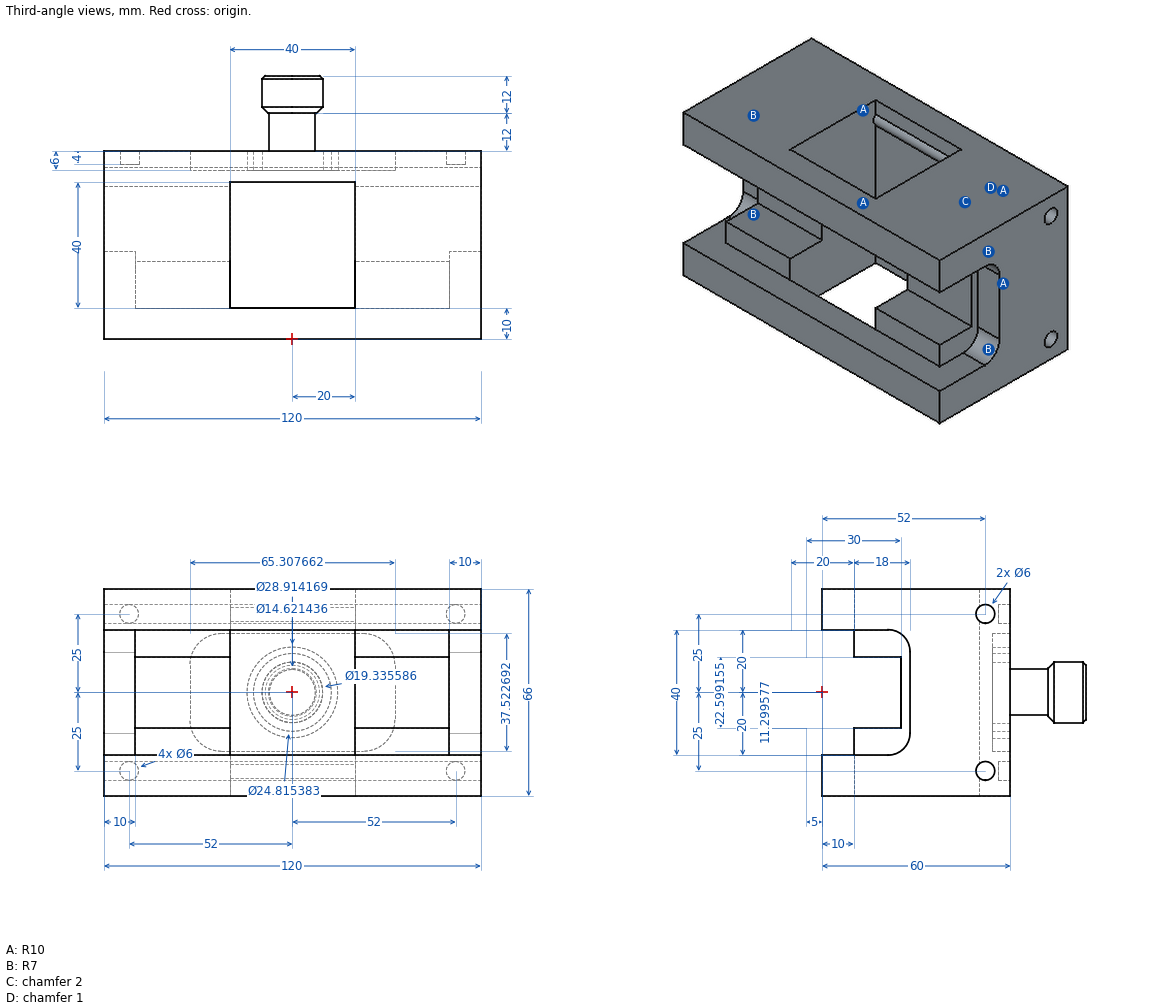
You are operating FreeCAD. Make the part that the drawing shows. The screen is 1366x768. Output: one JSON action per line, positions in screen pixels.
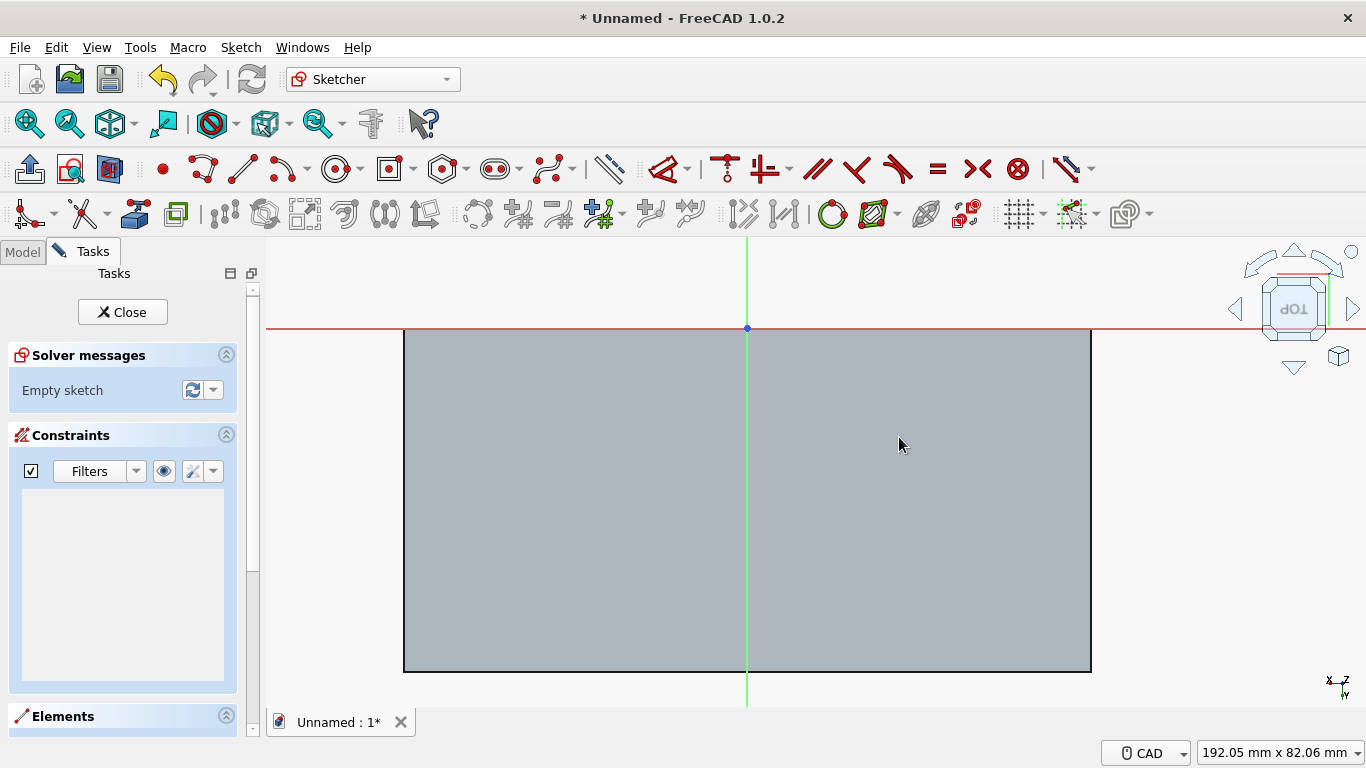
{"action": "key", "text": "g r"}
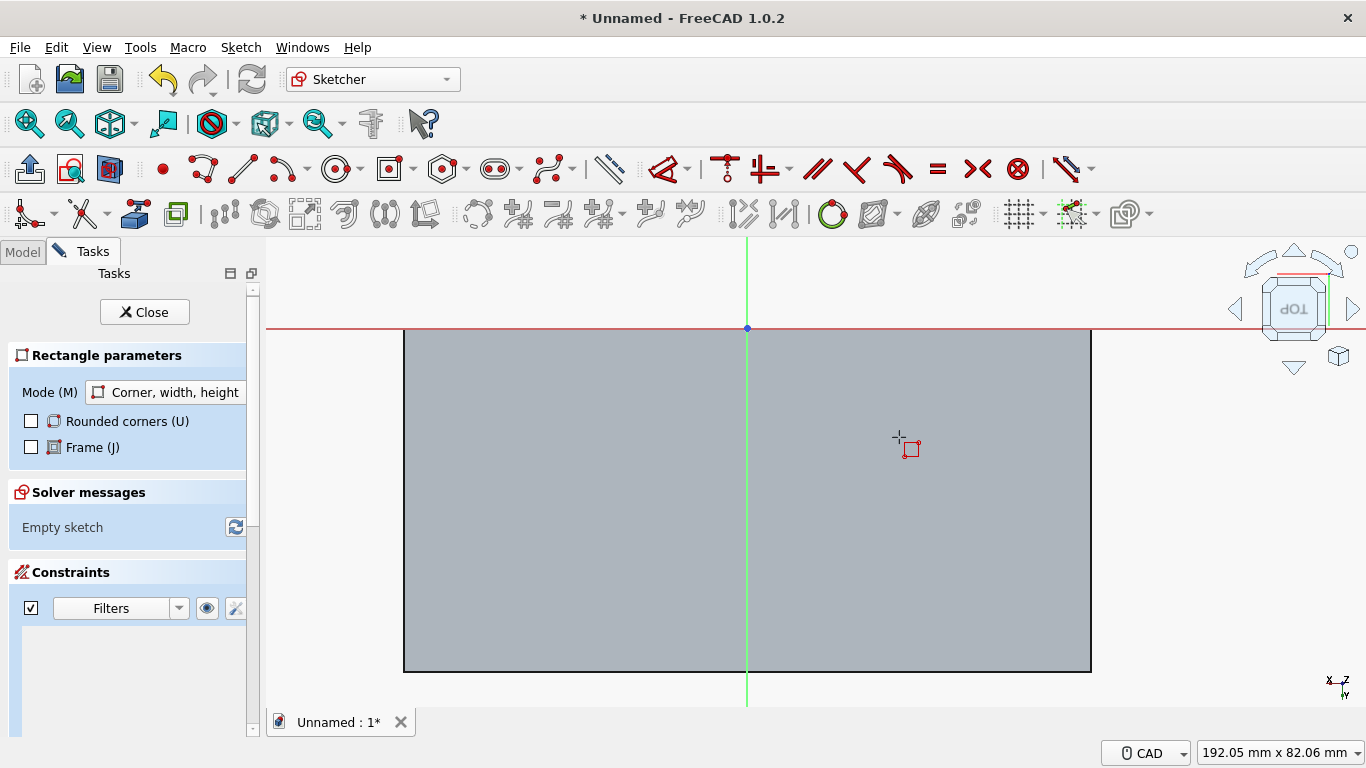
{"action": "left_click", "coordinate": [633, 386]}
{"action": "mouse_move", "coordinate": [862, 615]}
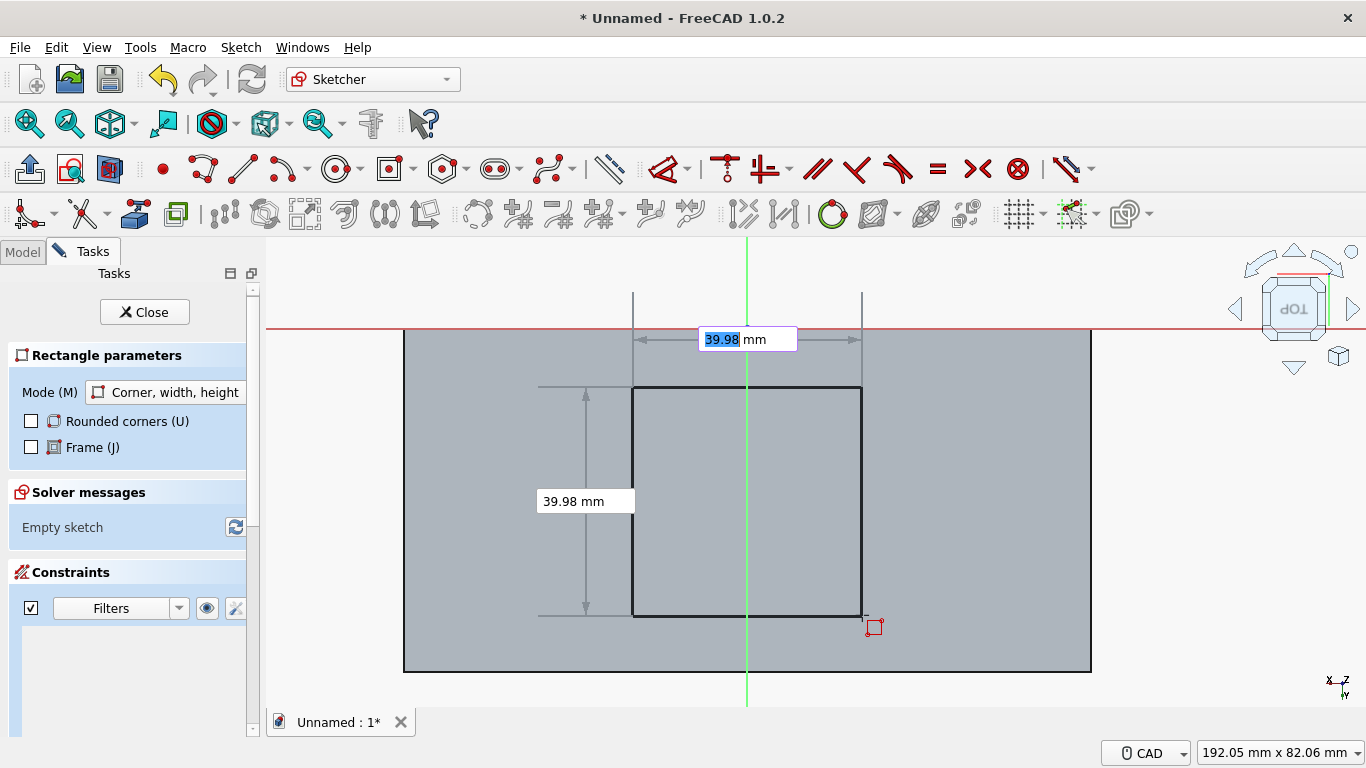
{"action": "type", "text": "40"}
{"action": "key", "text": "Tab"}
{"action": "type", "text": "40"}
{"action": "key", "text": "Return"}
{"action": "key", "text": "Escape"}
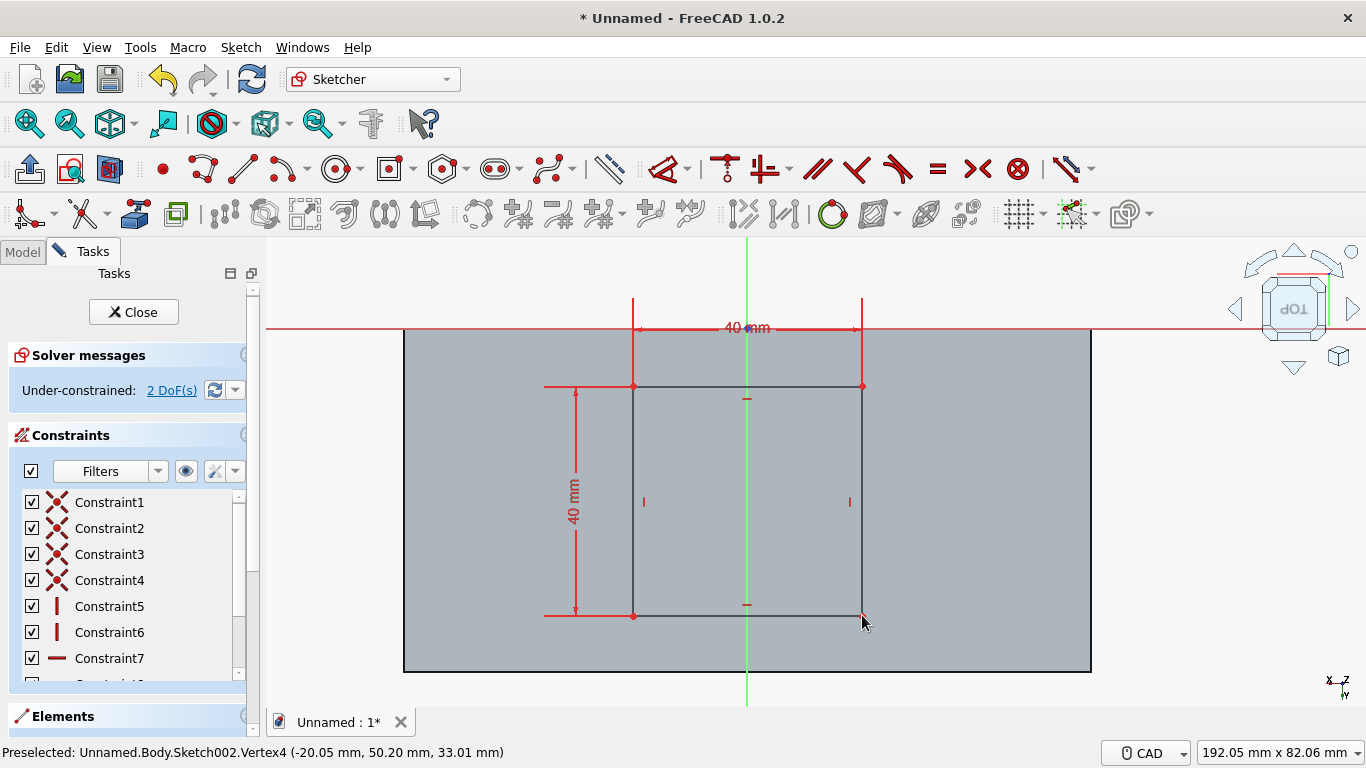
{"action": "left_click", "coordinate": [664, 170]}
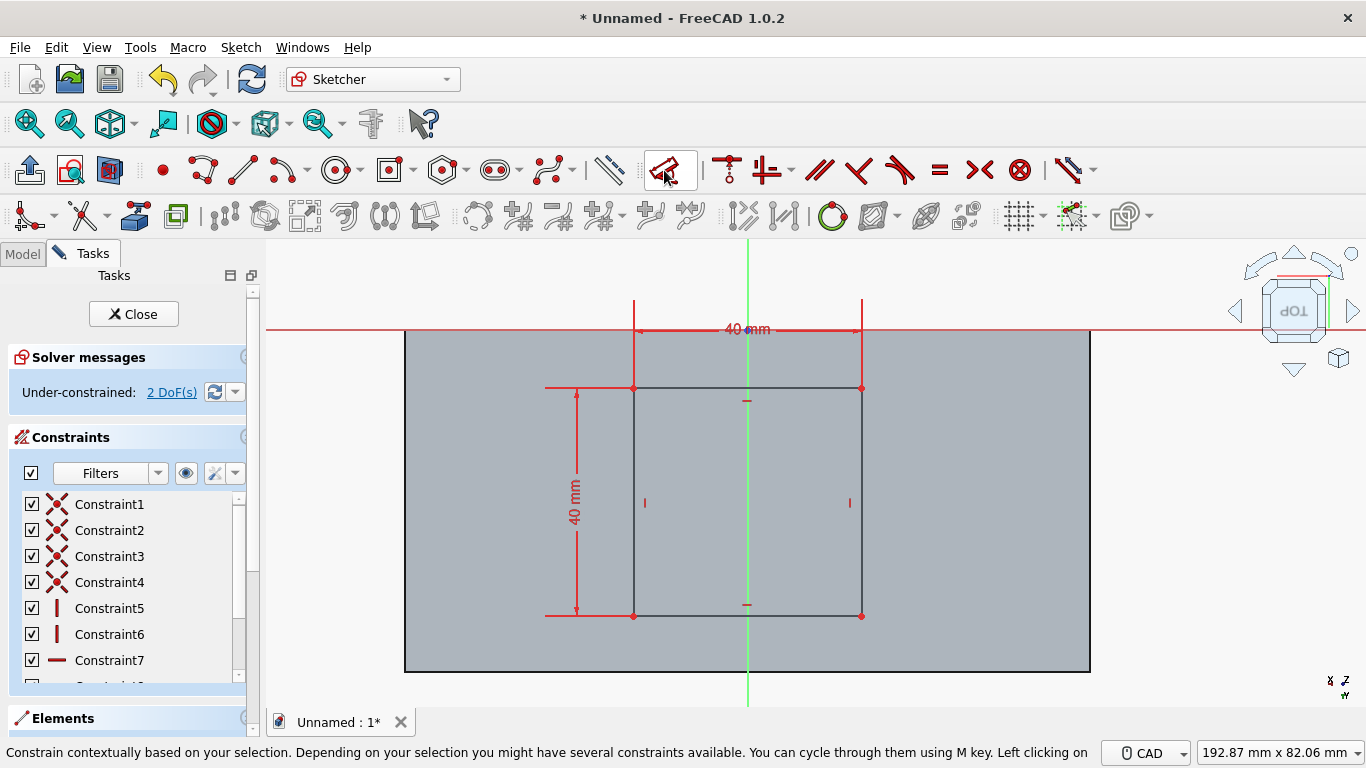
{"action": "left_click", "coordinate": [634, 388]}
{"action": "left_click", "coordinate": [691, 296]}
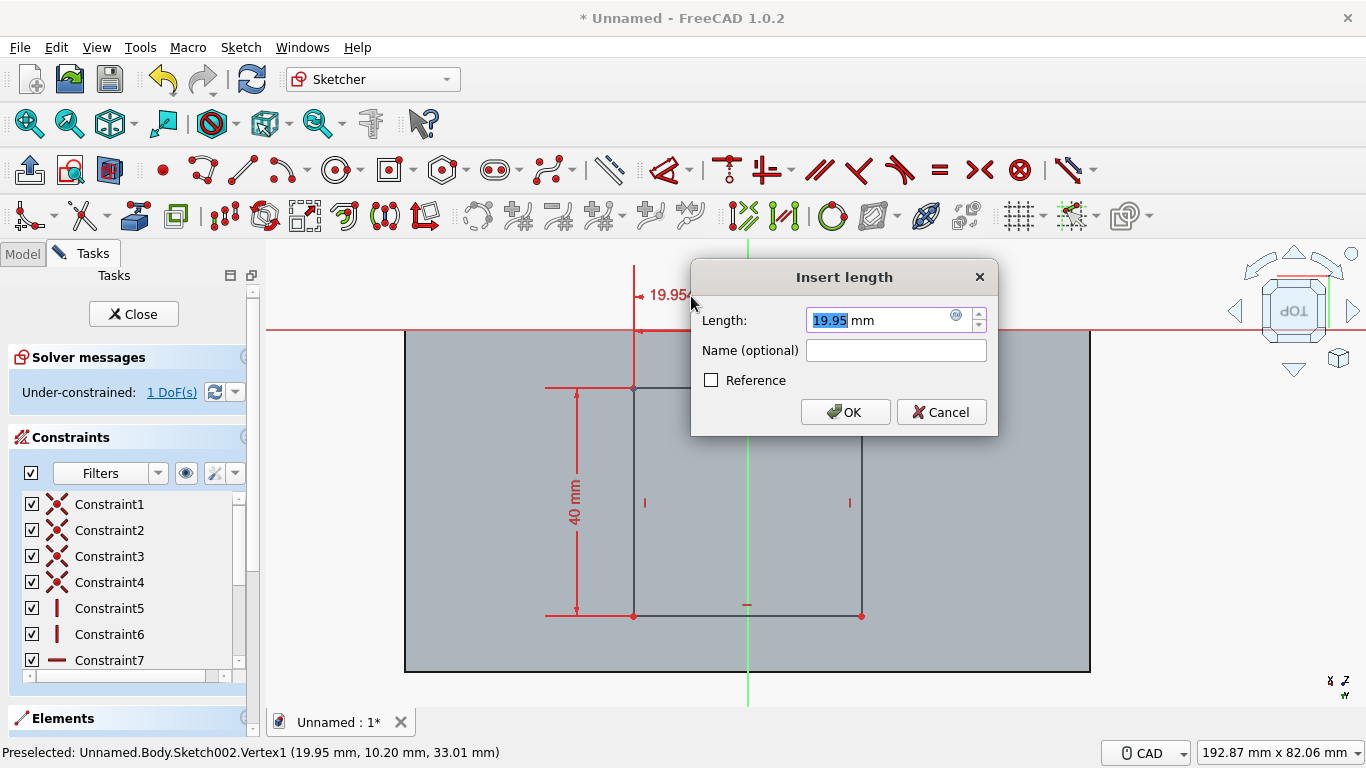
{"action": "type", "text": "20"}
{"action": "key", "text": "Return"}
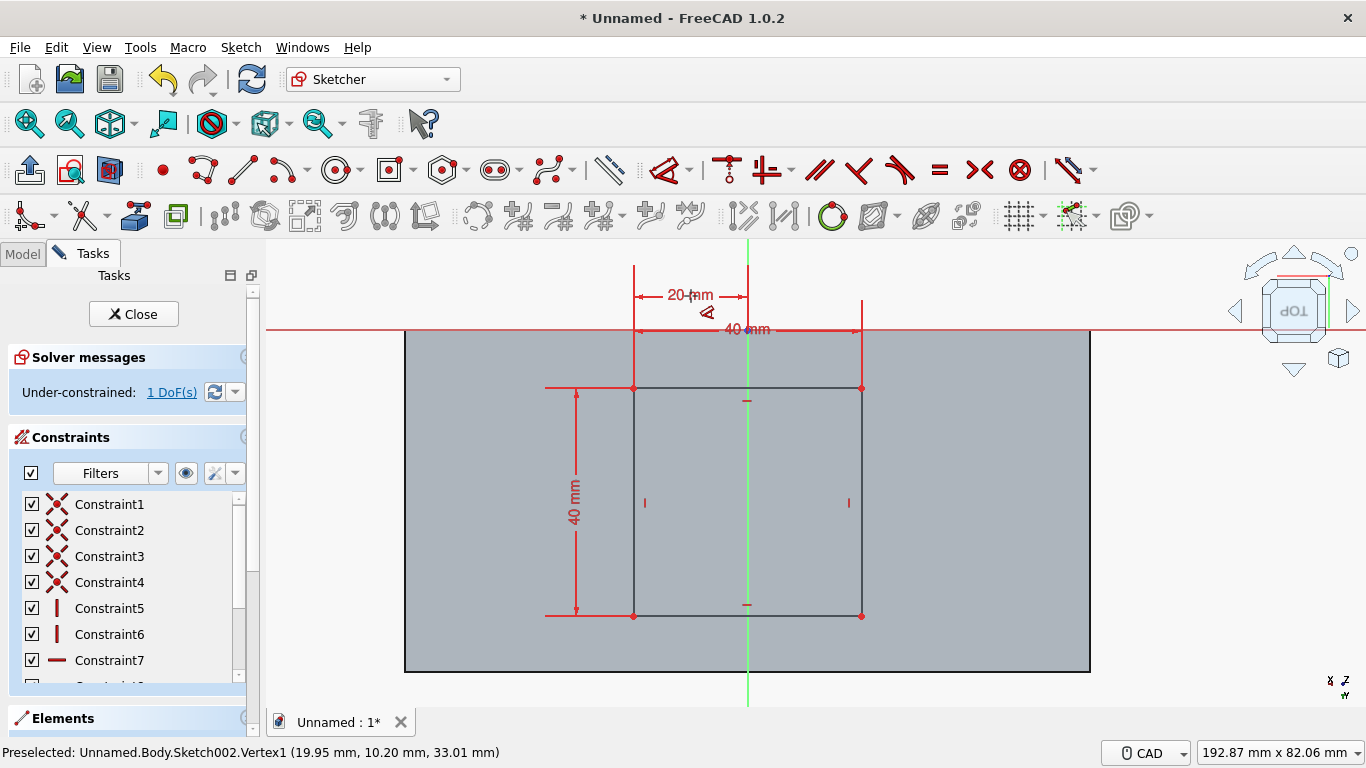
{"action": "left_click", "coordinate": [634, 388]}
{"action": "left_click", "coordinate": [600, 359]}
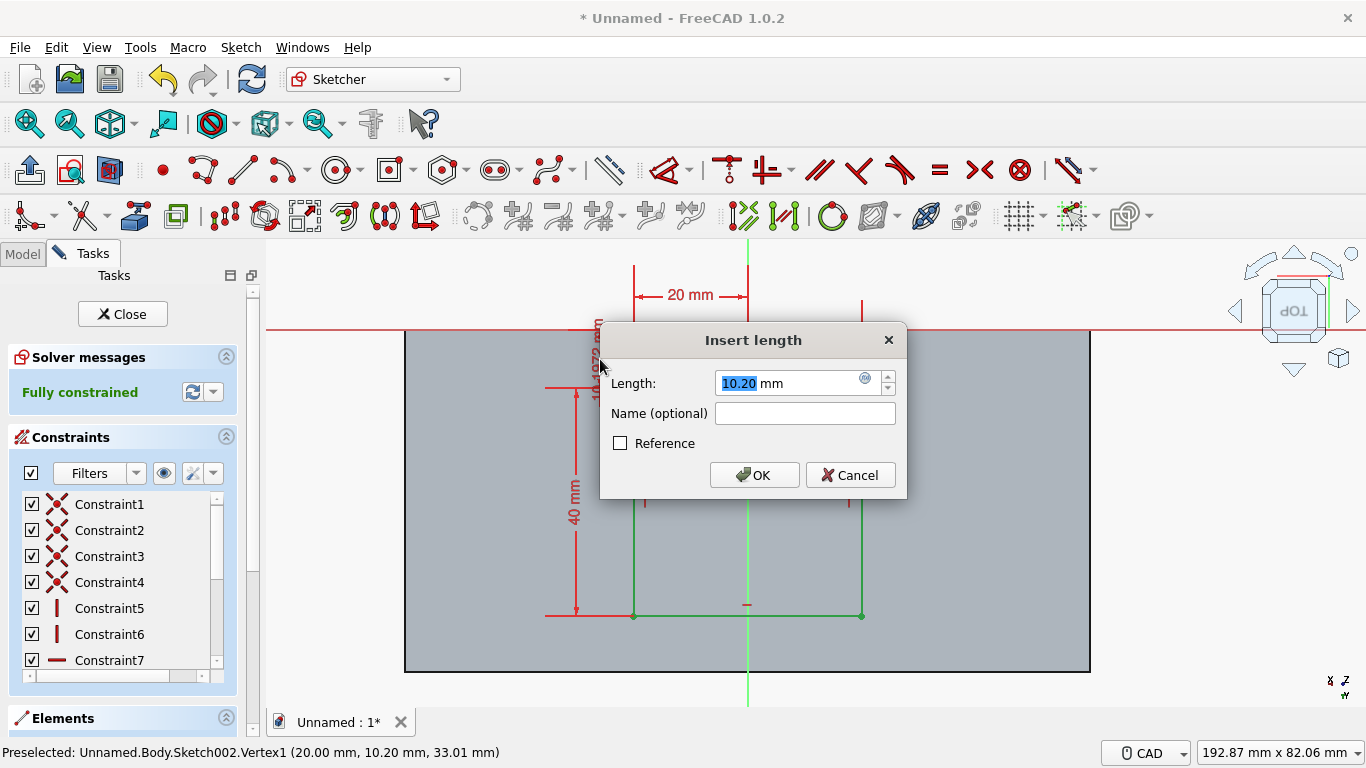
{"action": "type", "text": "10"}
{"action": "key", "text": "Return"}
{"action": "key", "text": "Escape"}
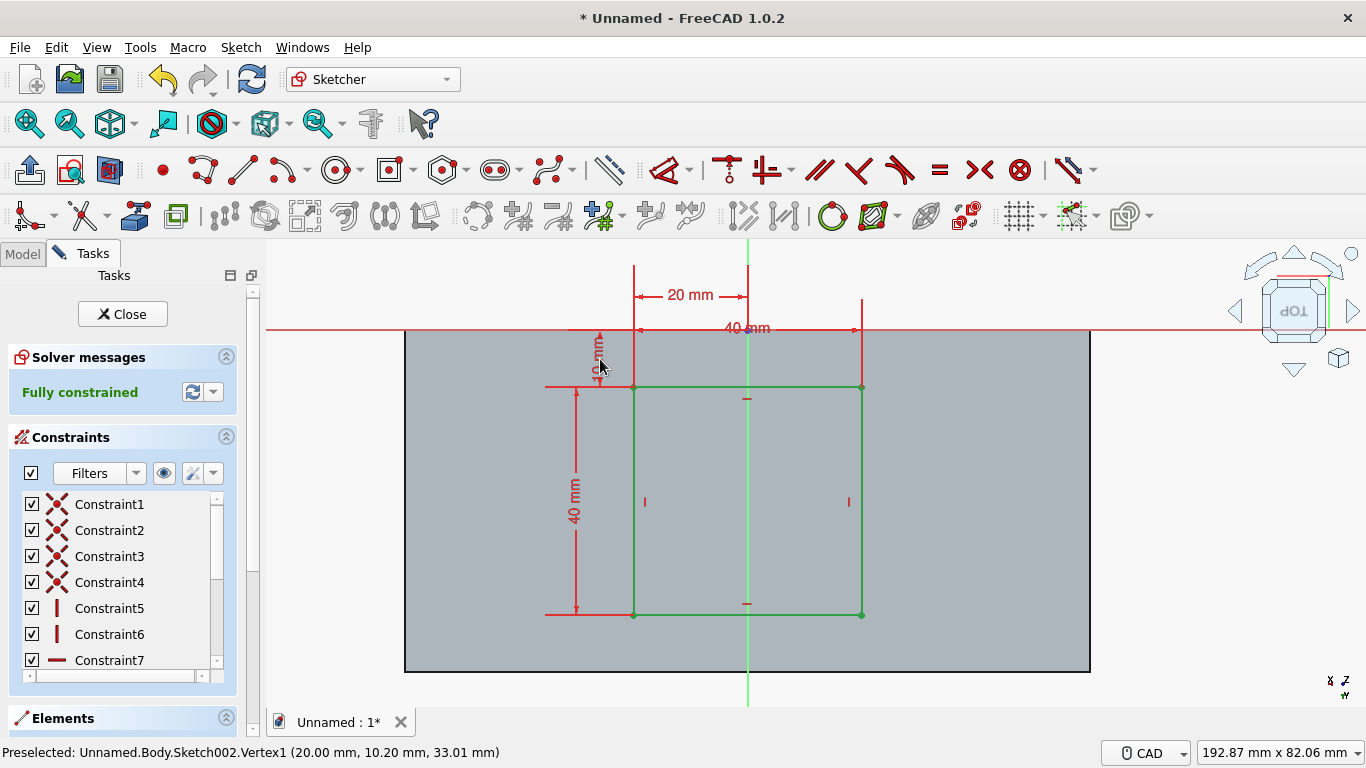
{"action": "left_click", "coordinate": [123, 314]}